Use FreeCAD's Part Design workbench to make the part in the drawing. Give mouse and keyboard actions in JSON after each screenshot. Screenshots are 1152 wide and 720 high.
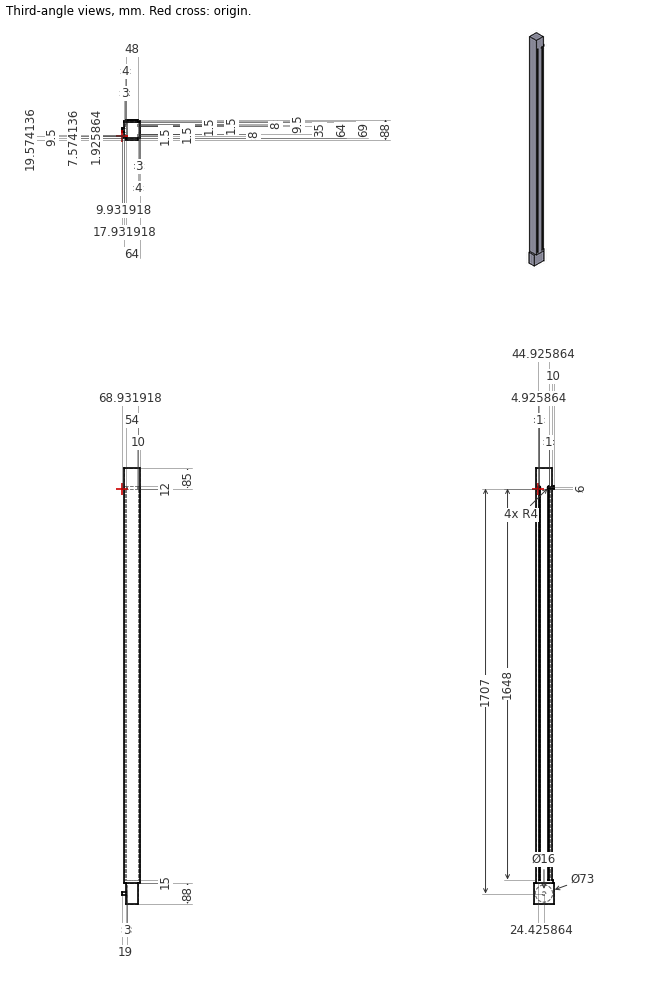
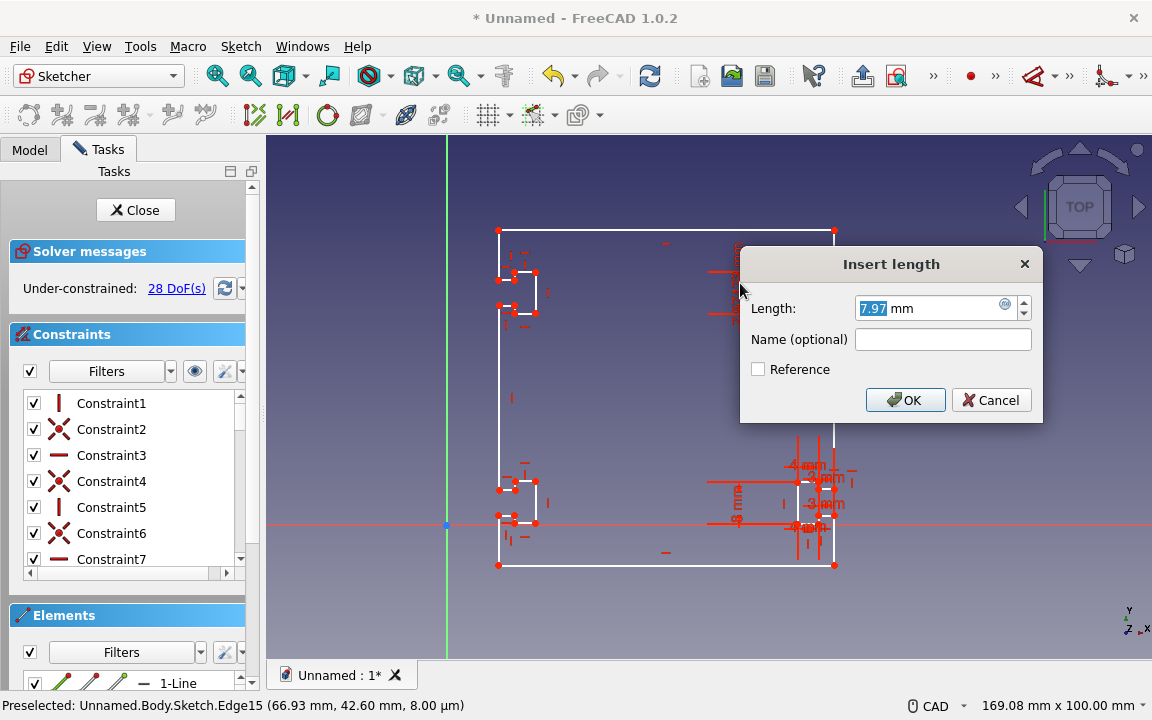
{"action": "type", "text": "8"}
{"action": "key", "text": "Return"}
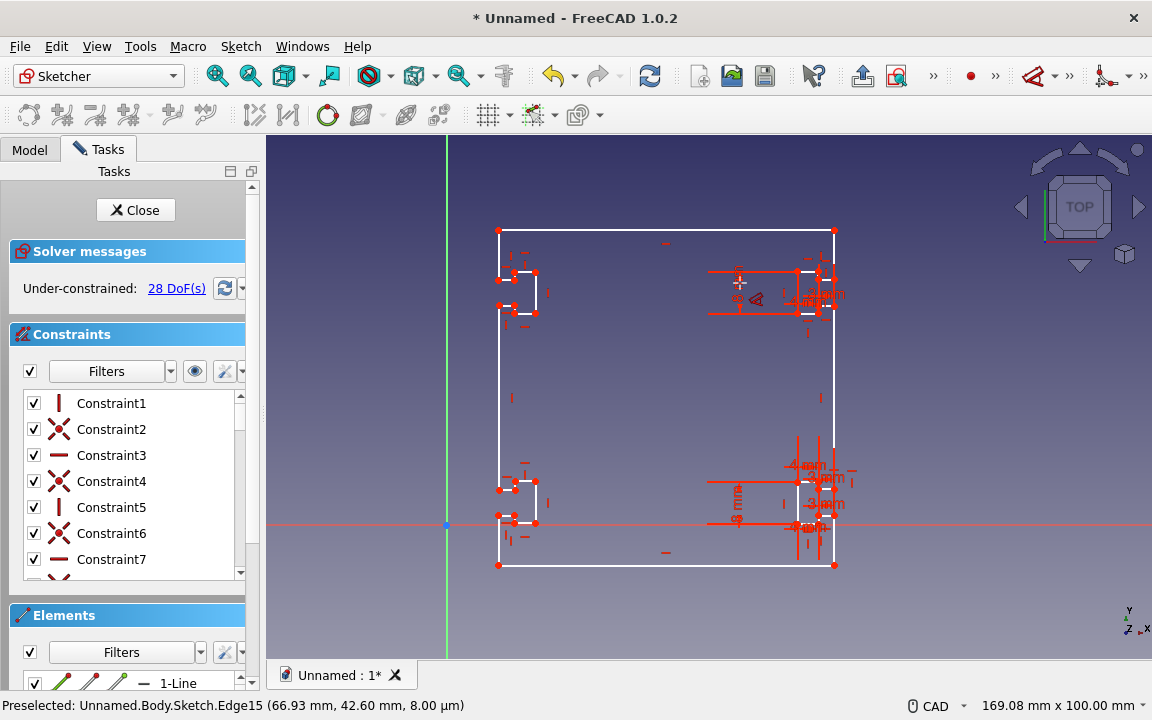
{"action": "scroll", "coordinate": [808, 272], "scroll_direction": "up", "scroll_amount": 4}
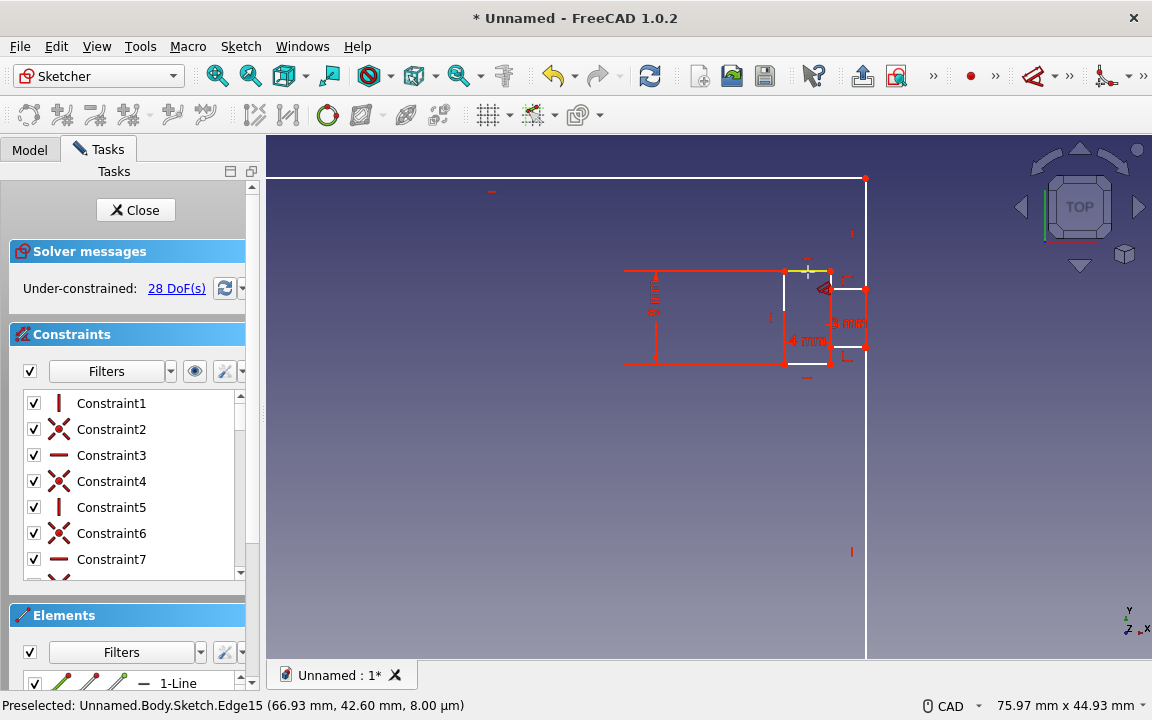
{"action": "left_click", "coordinate": [807, 271]}
{"action": "left_click", "coordinate": [807, 237]}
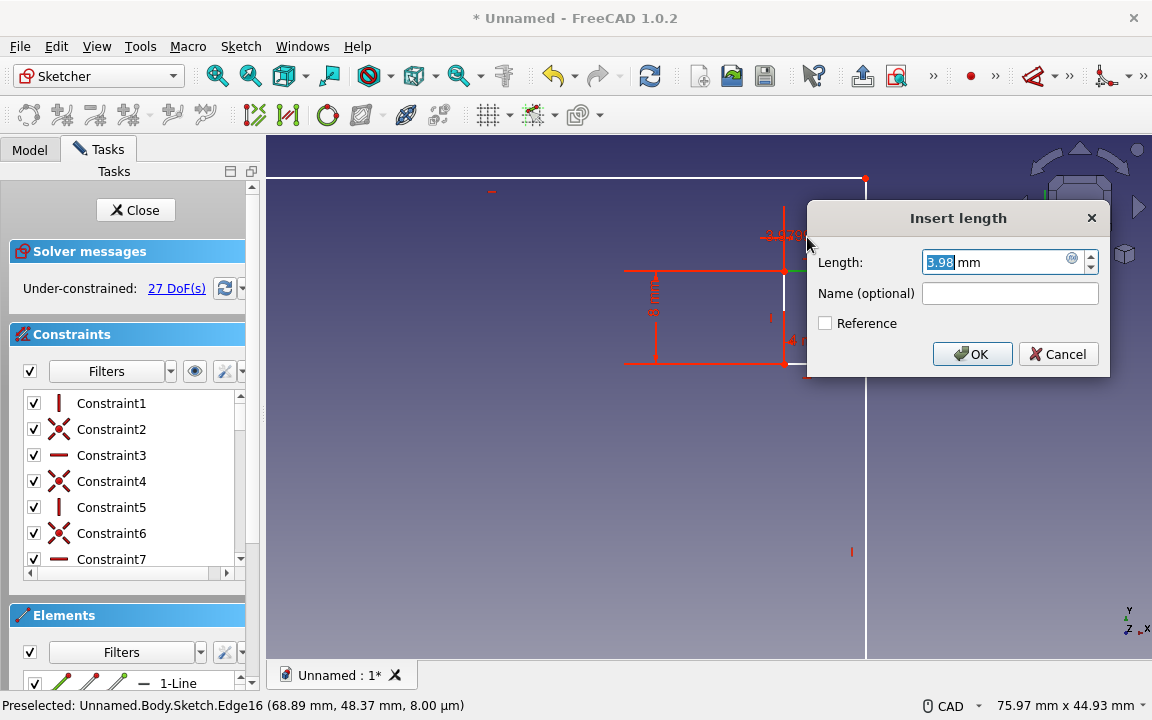
{"action": "type", "text": "4"}
{"action": "key", "text": "Return"}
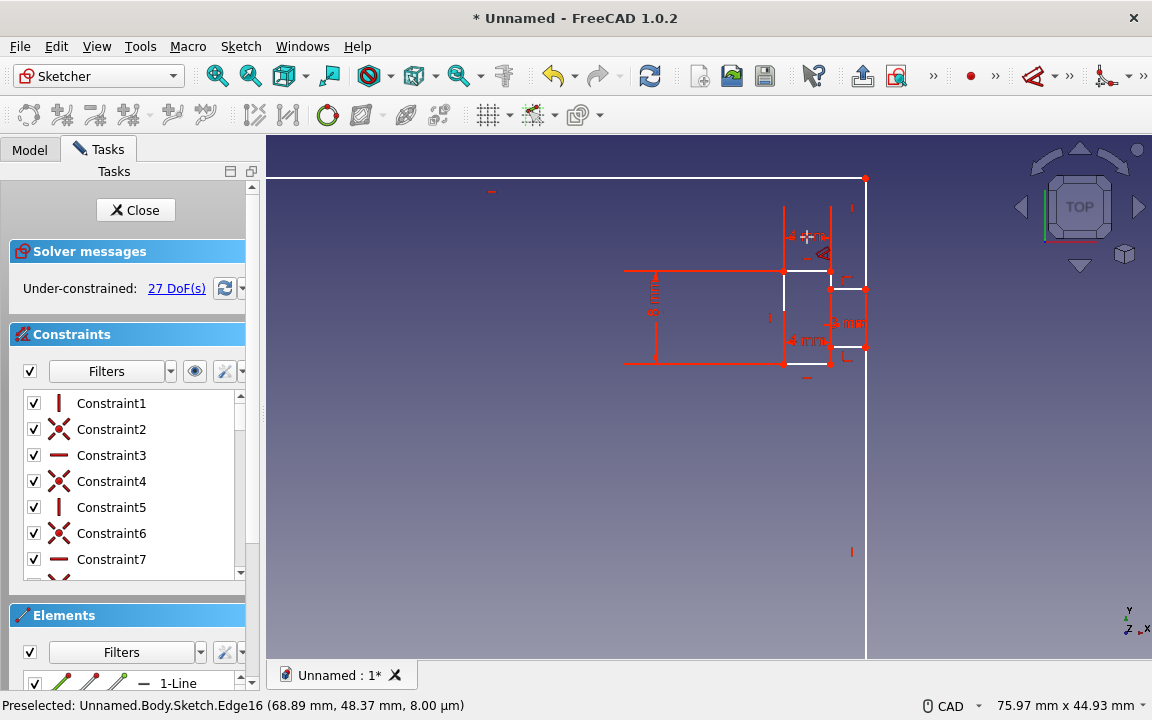
{"action": "scroll", "coordinate": [841, 289], "scroll_direction": "up", "scroll_amount": 2}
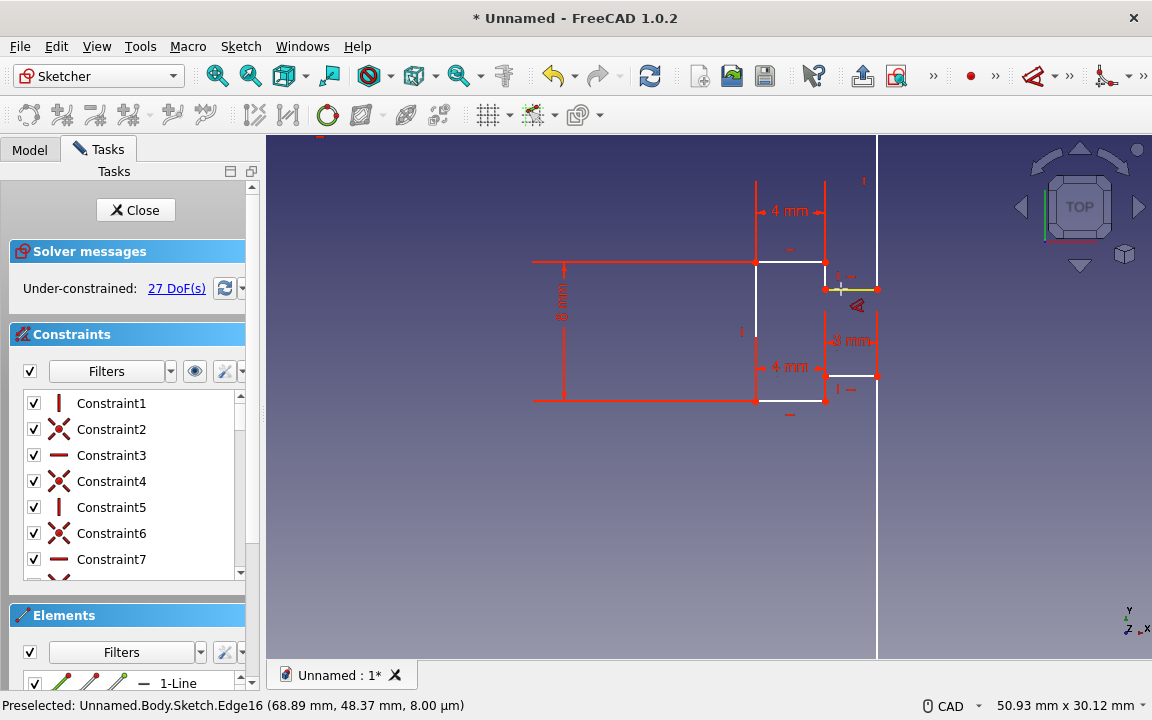
{"action": "left_click", "coordinate": [841, 290]}
{"action": "left_click", "coordinate": [851, 256]}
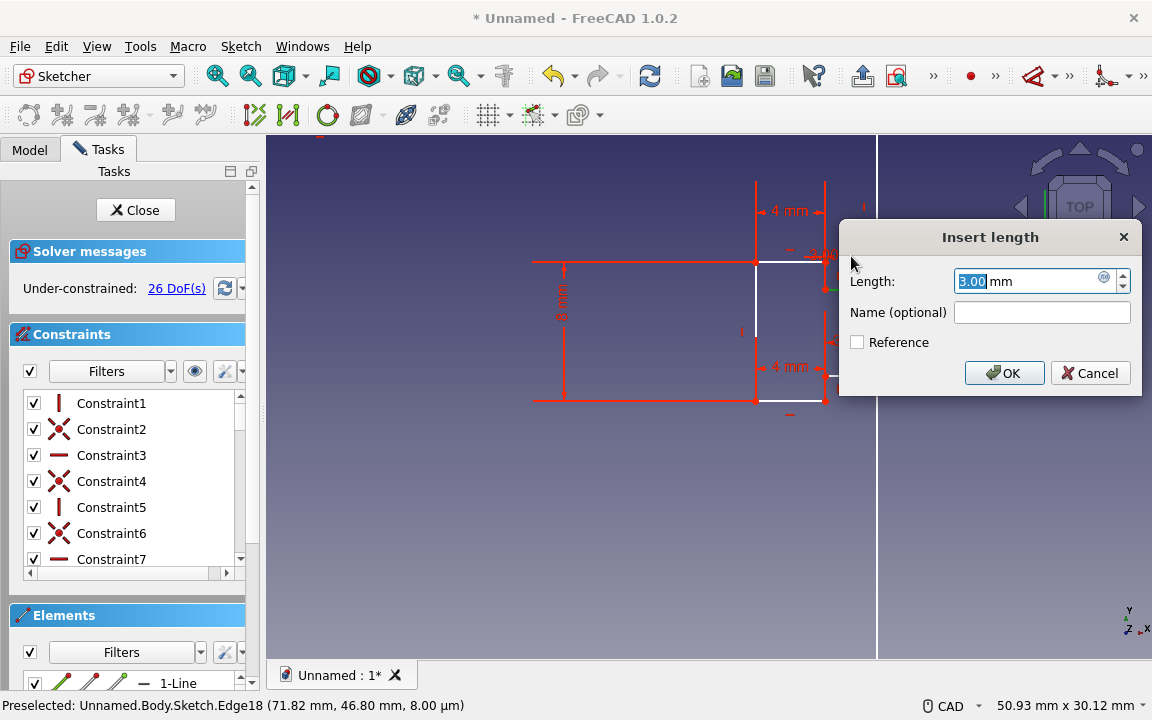
{"action": "type", "text": "3"}
{"action": "key", "text": "Return"}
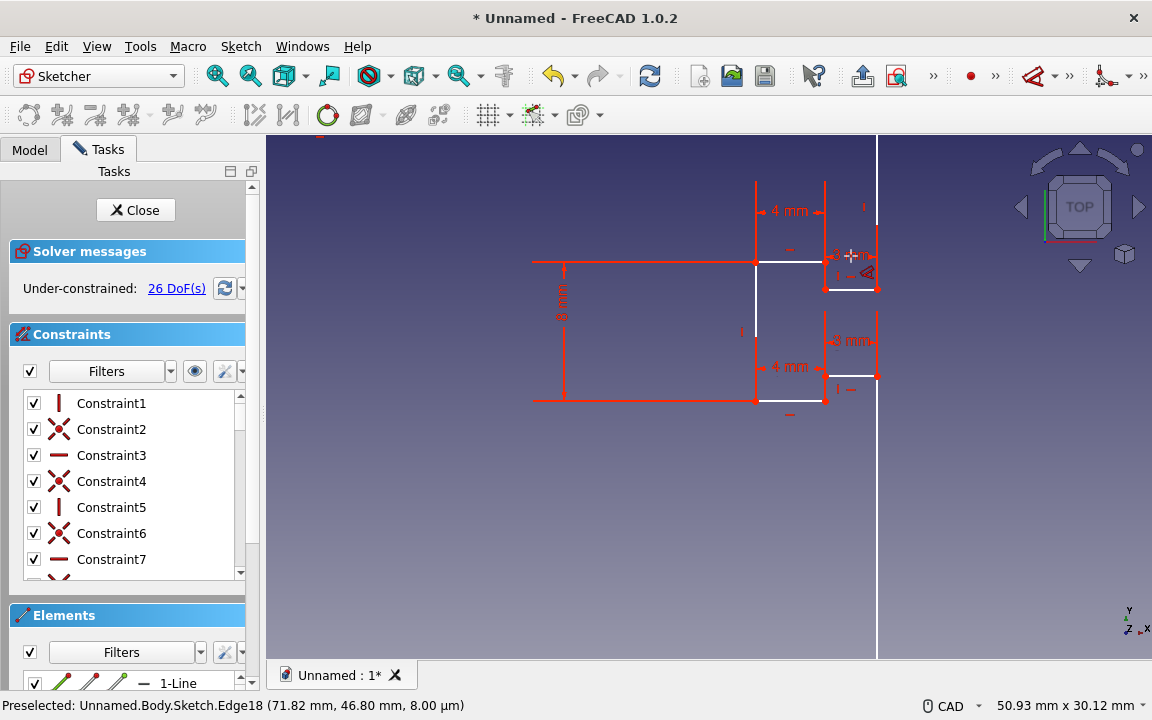
{"action": "scroll", "coordinate": [815, 276], "scroll_direction": "down", "scroll_amount": 6}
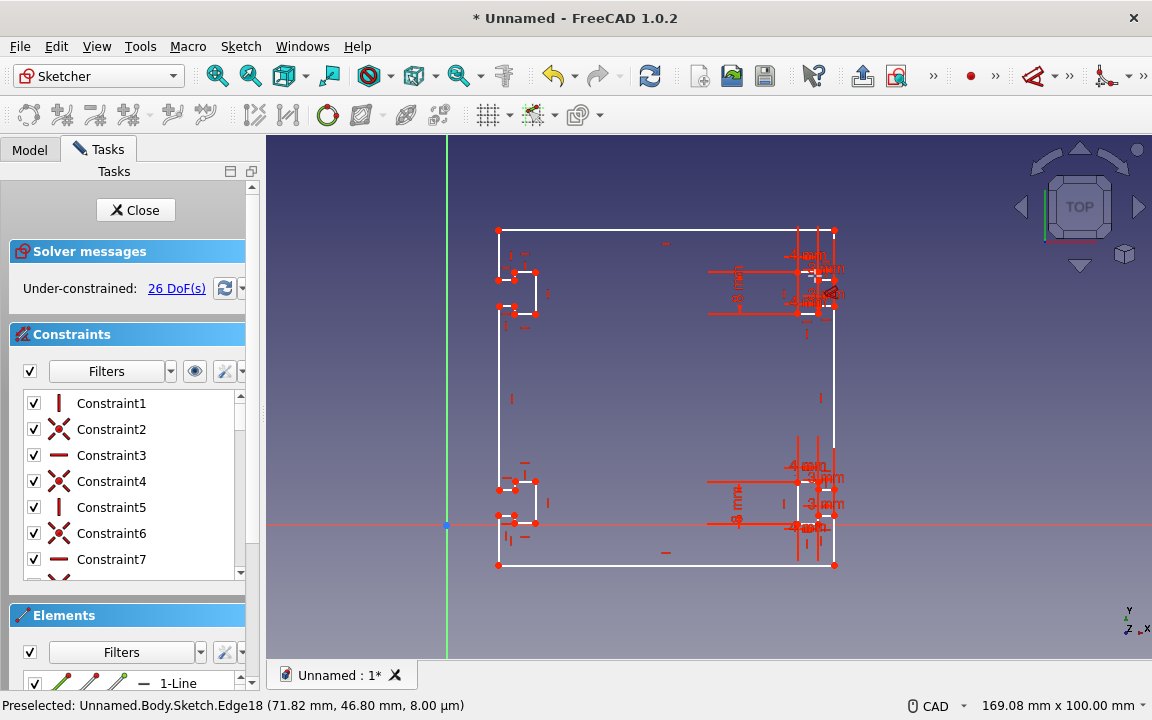
{"action": "scroll", "coordinate": [503, 280], "scroll_direction": "up", "scroll_amount": 6}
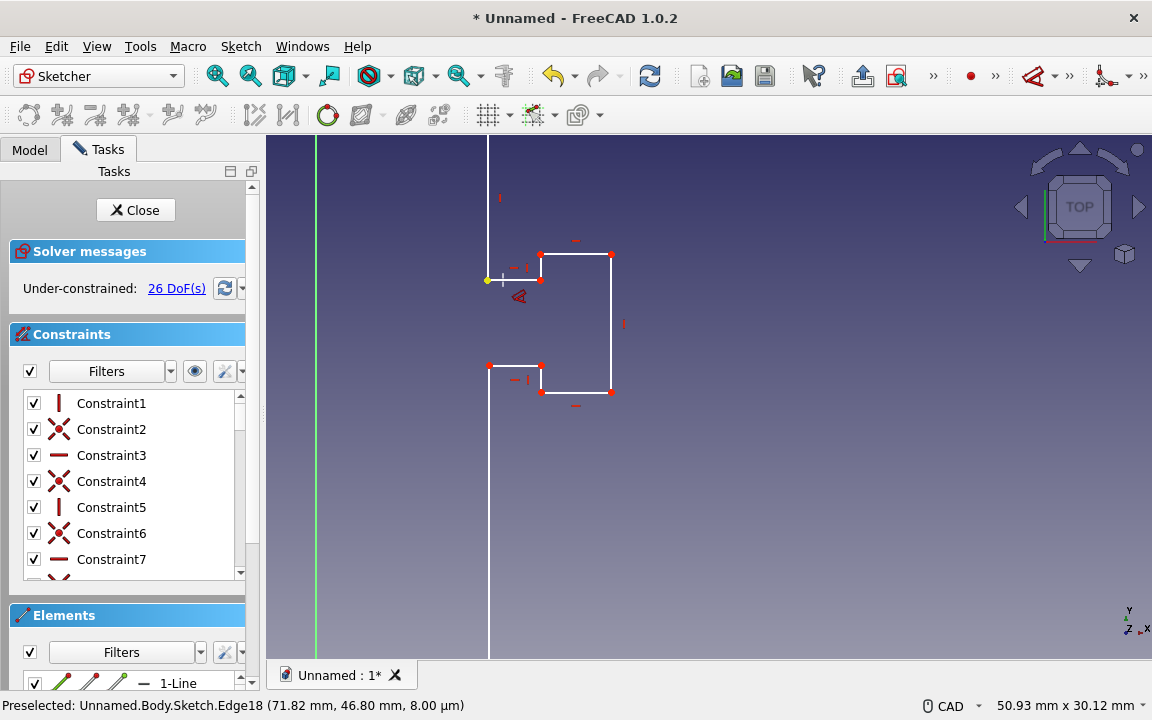
{"action": "left_click", "coordinate": [504, 280]}
{"action": "left_click", "coordinate": [514, 246]}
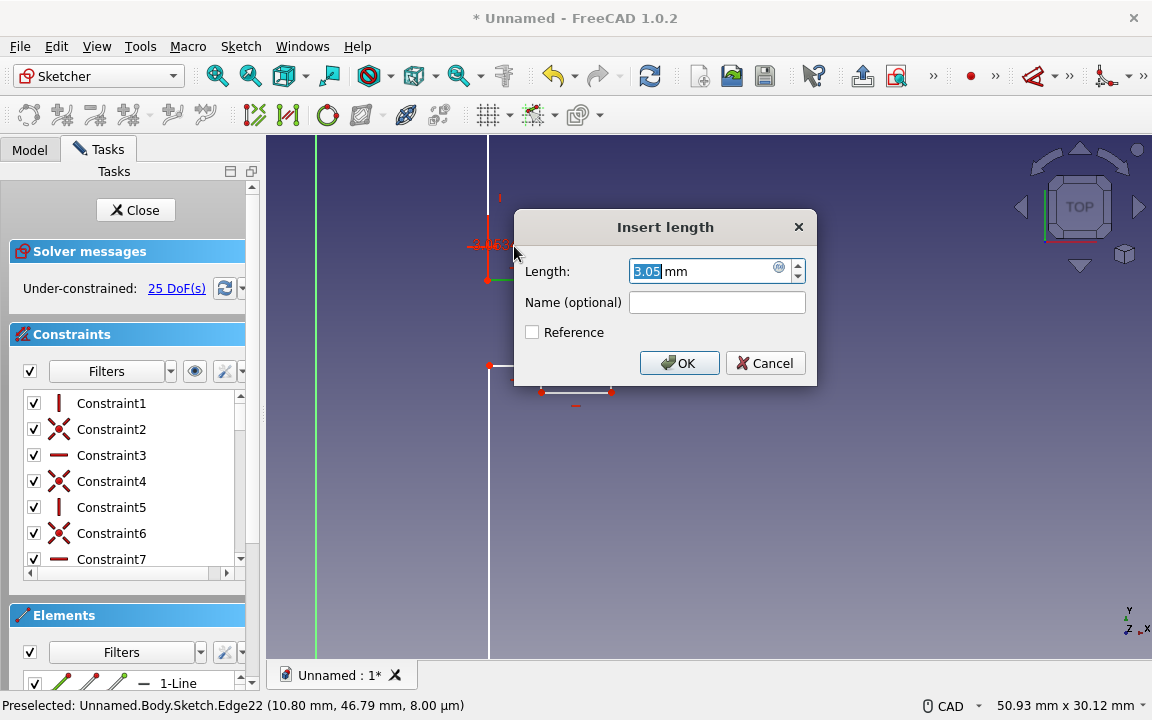
{"action": "type", "text": "3"}
{"action": "key", "text": "Return"}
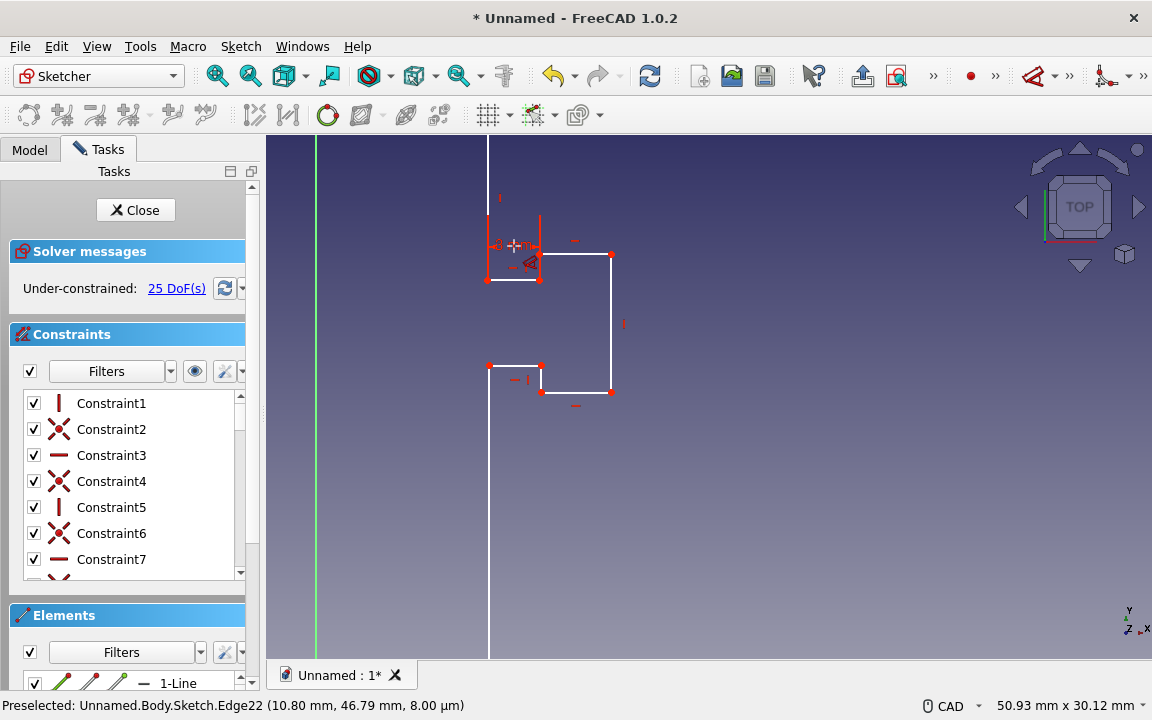
{"action": "left_click", "coordinate": [561, 254]}
{"action": "left_click", "coordinate": [576, 220]}